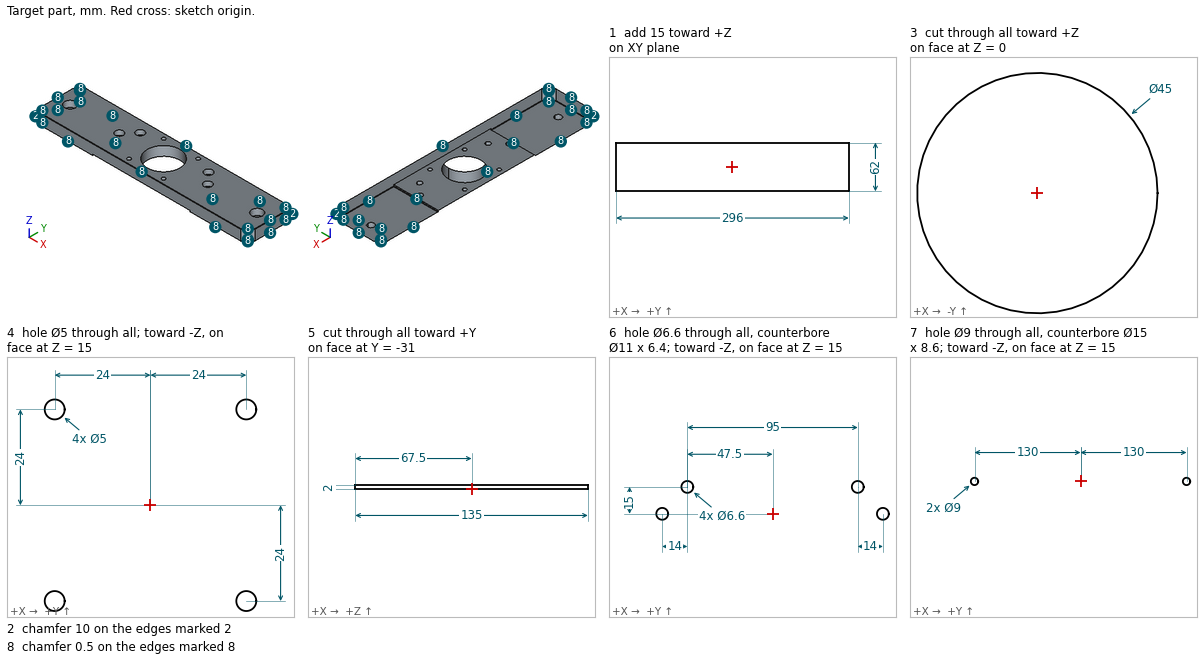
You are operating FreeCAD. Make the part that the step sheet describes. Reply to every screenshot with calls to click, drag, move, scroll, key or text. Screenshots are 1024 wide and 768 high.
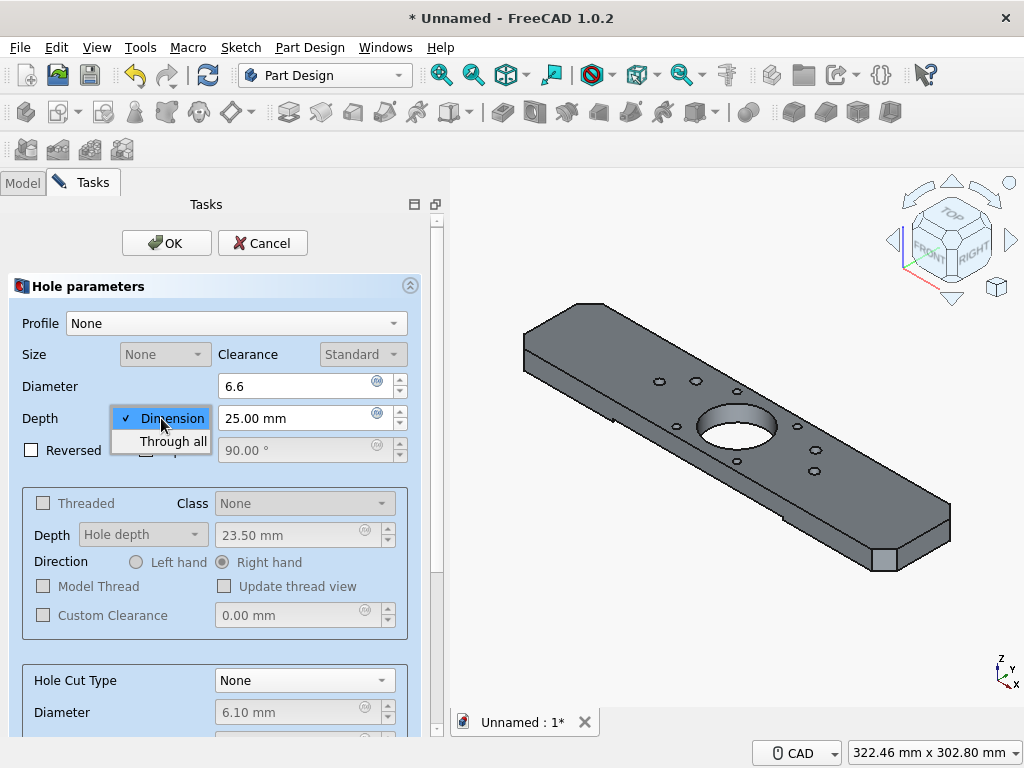
click(160, 442)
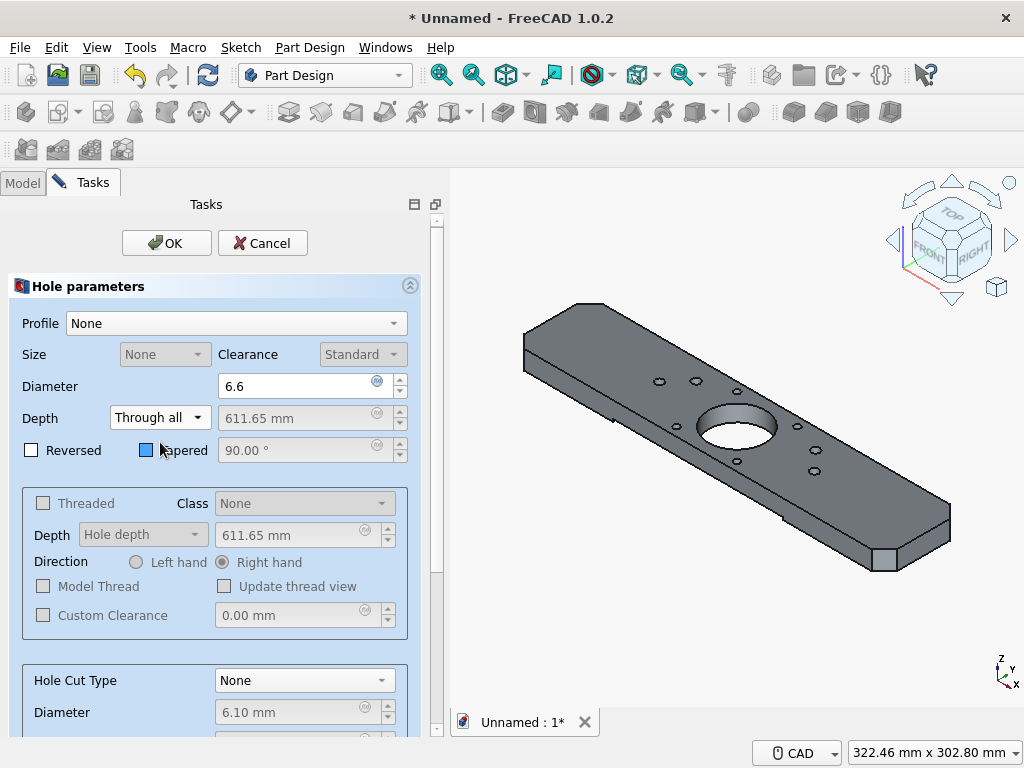
click(306, 680)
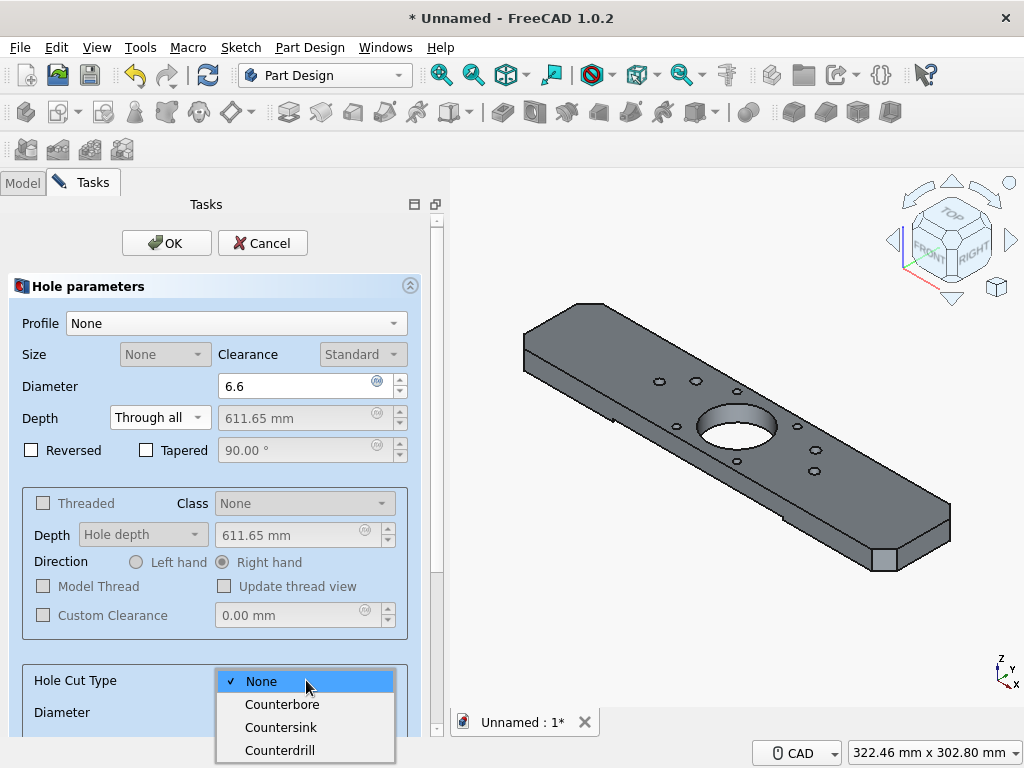
click(304, 704)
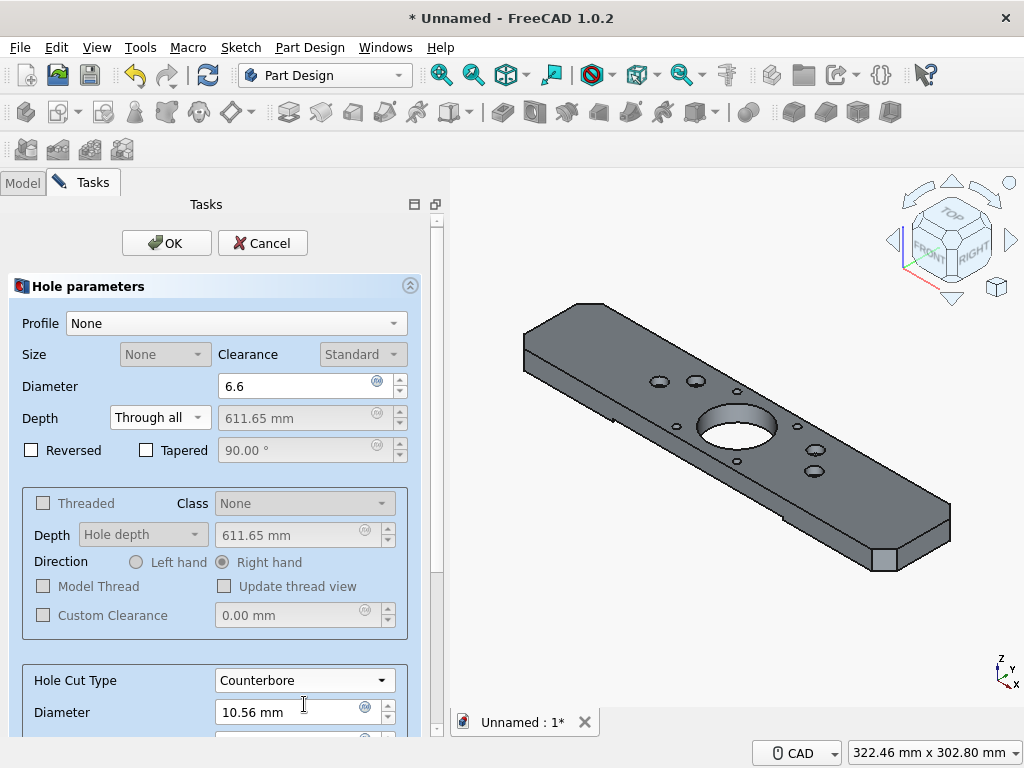
triple_click(298, 712)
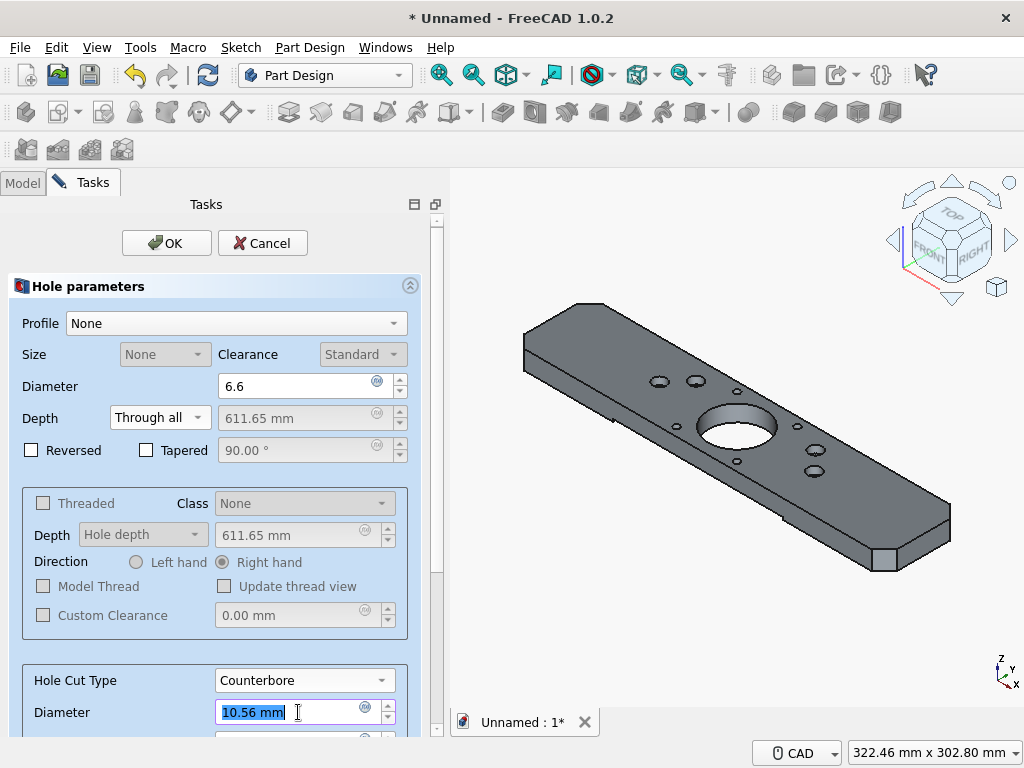
text(11)
key(Tab)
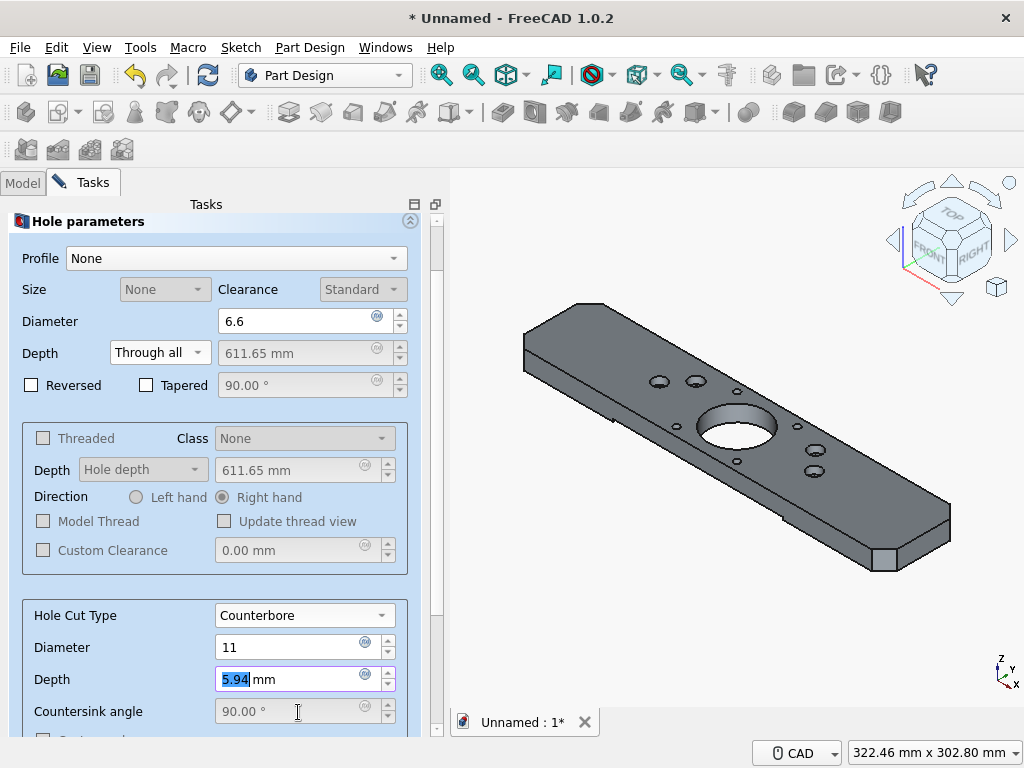
text(6.4)
key(Tab)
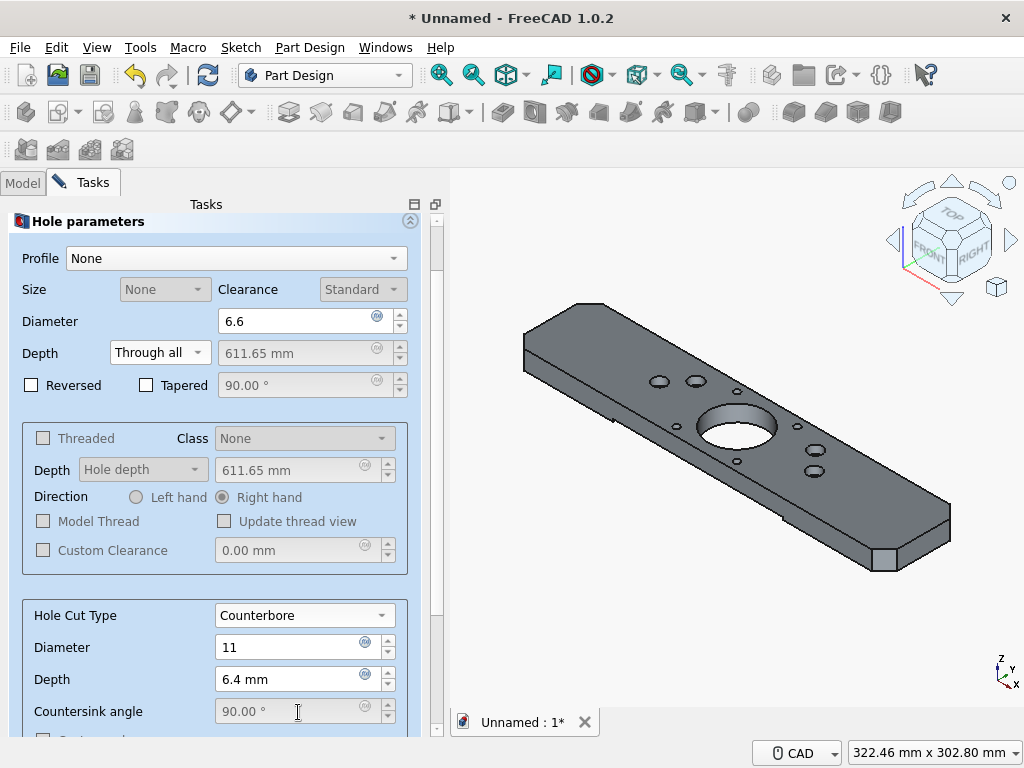
scroll(437, 475, up, 2)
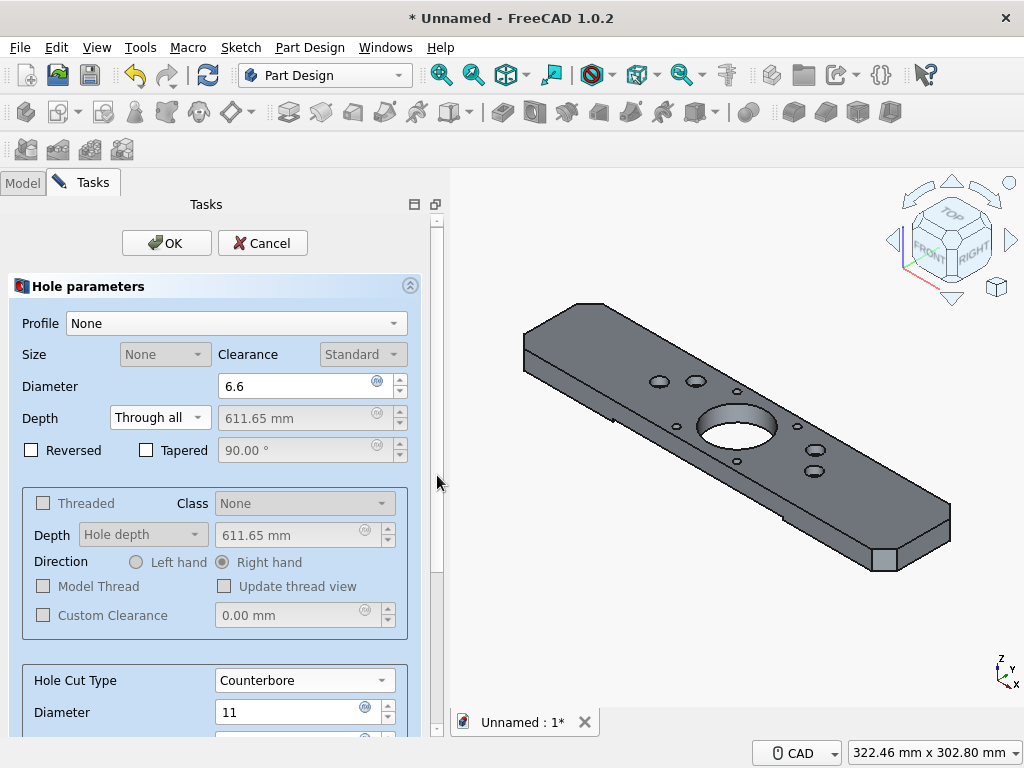
click(167, 243)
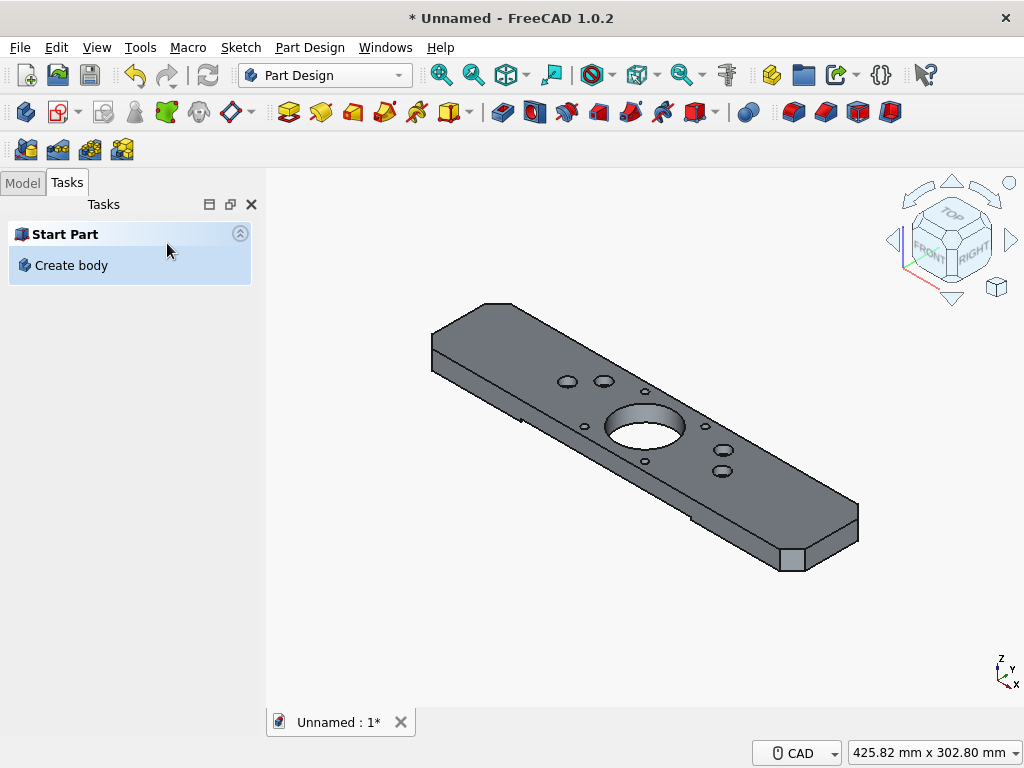
click(816, 511)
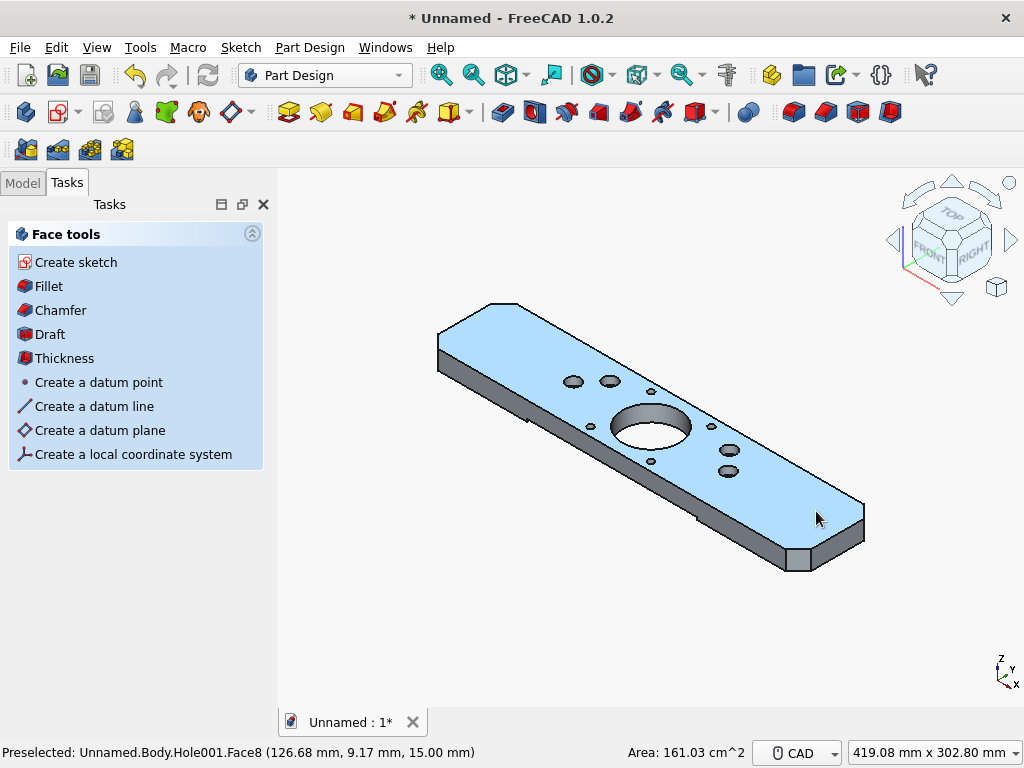
click(58, 112)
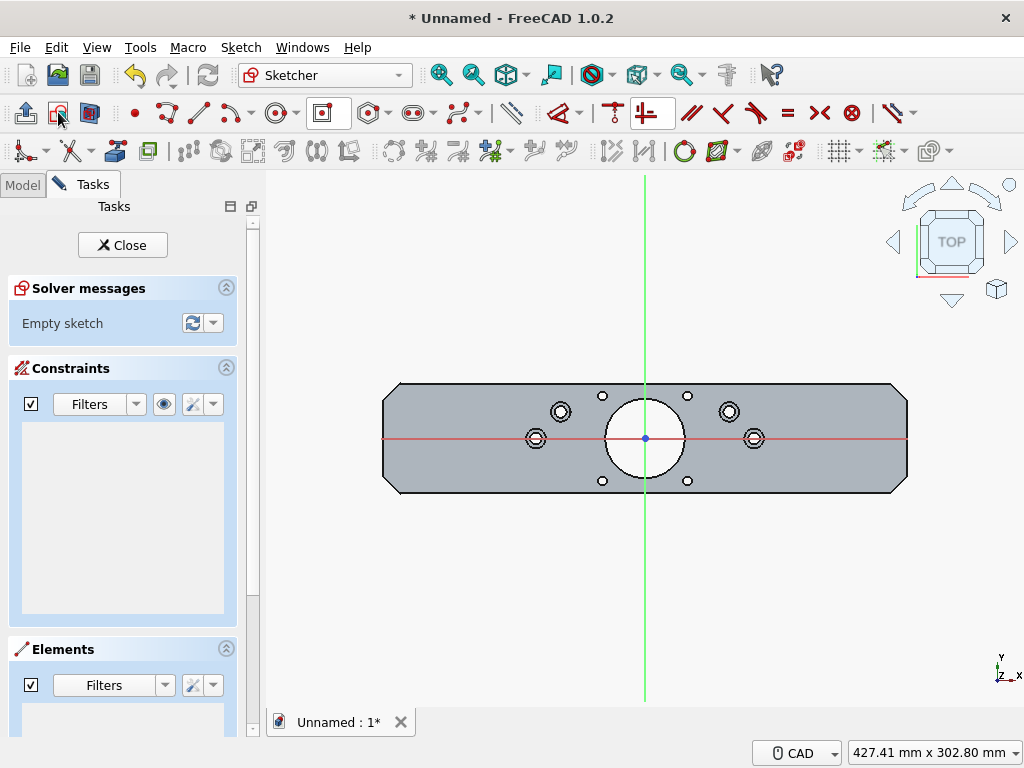
scroll(294, 439, down, 1)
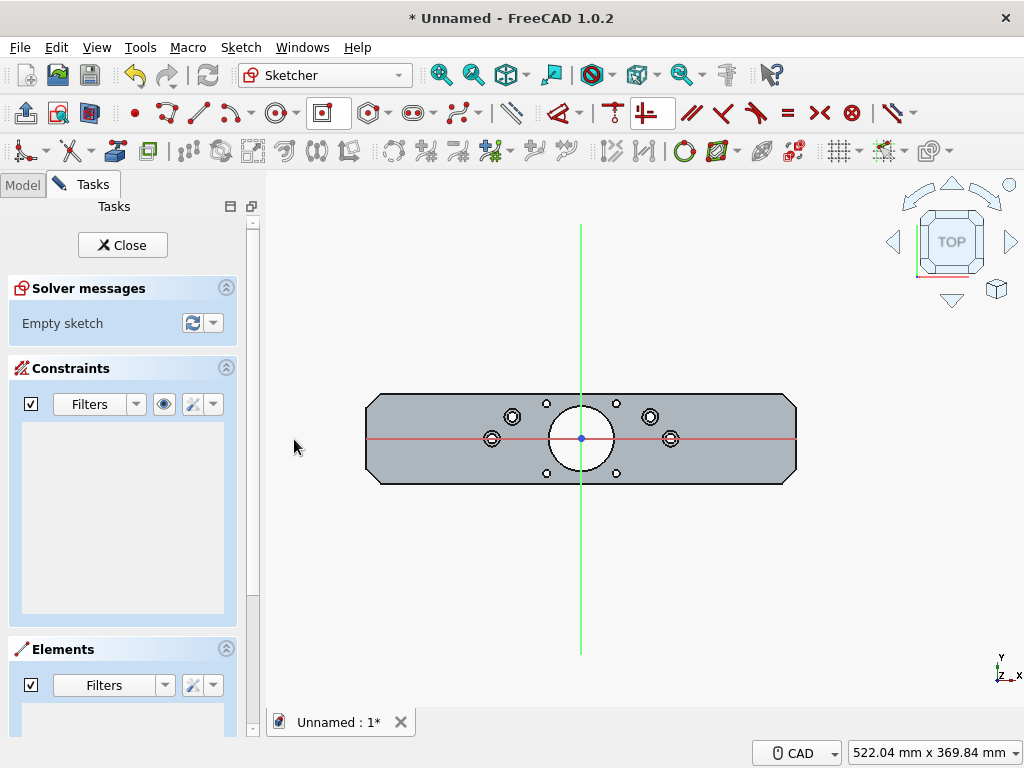
click(276, 114)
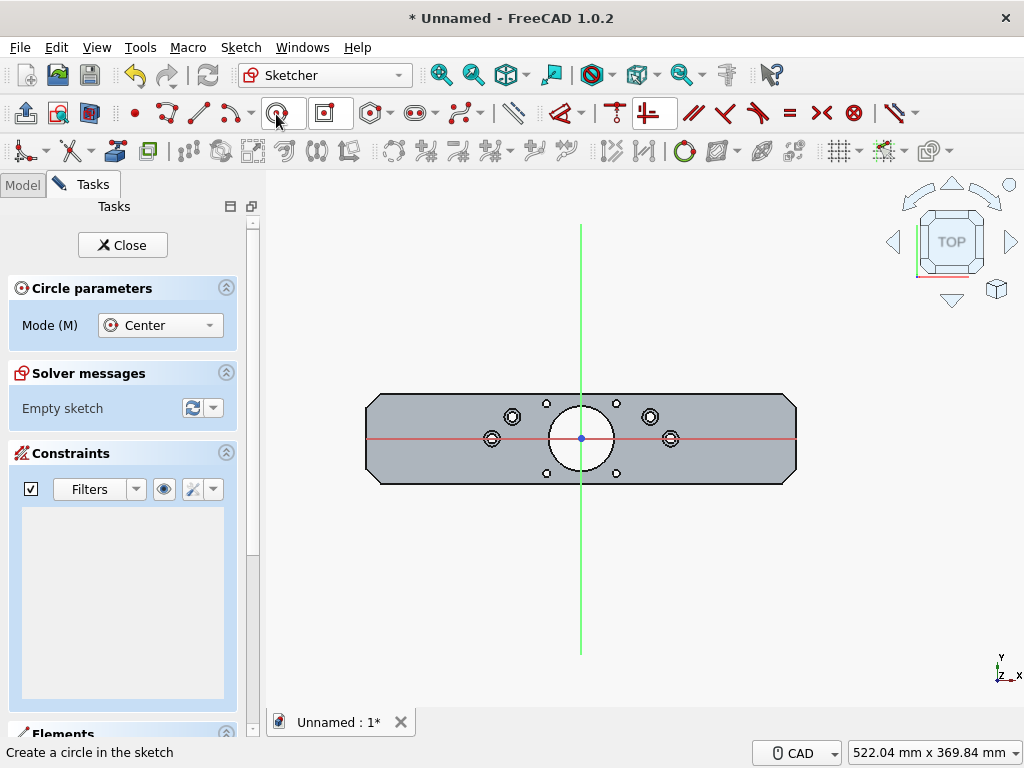
scroll(393, 439, up, 7)